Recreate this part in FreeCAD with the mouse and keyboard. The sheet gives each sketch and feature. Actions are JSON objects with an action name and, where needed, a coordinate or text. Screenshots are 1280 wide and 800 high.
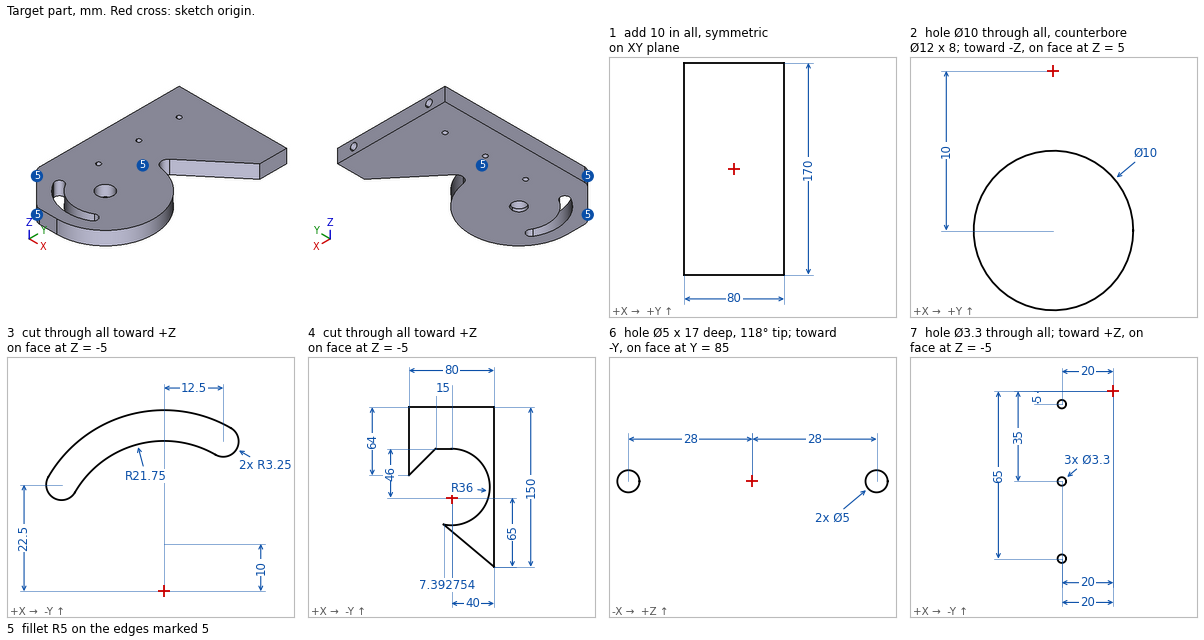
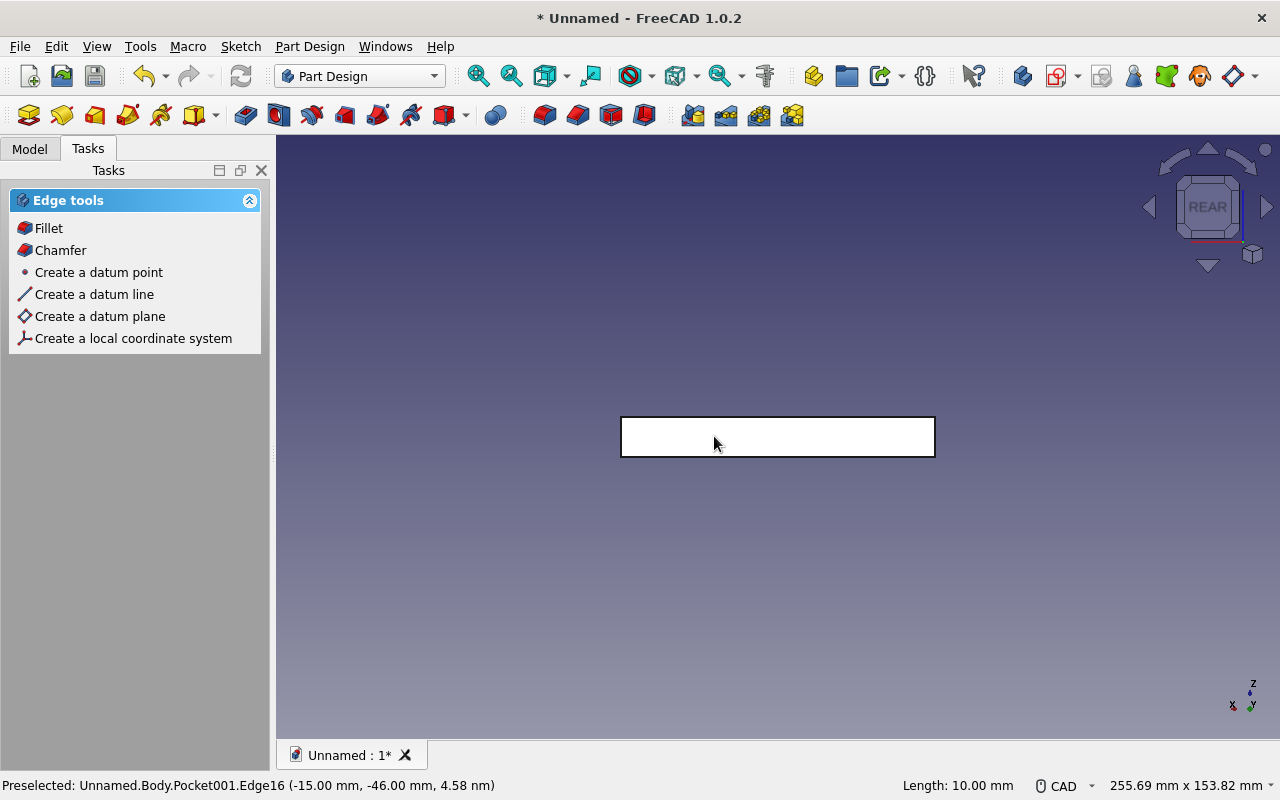
{"action": "key", "text": "6"}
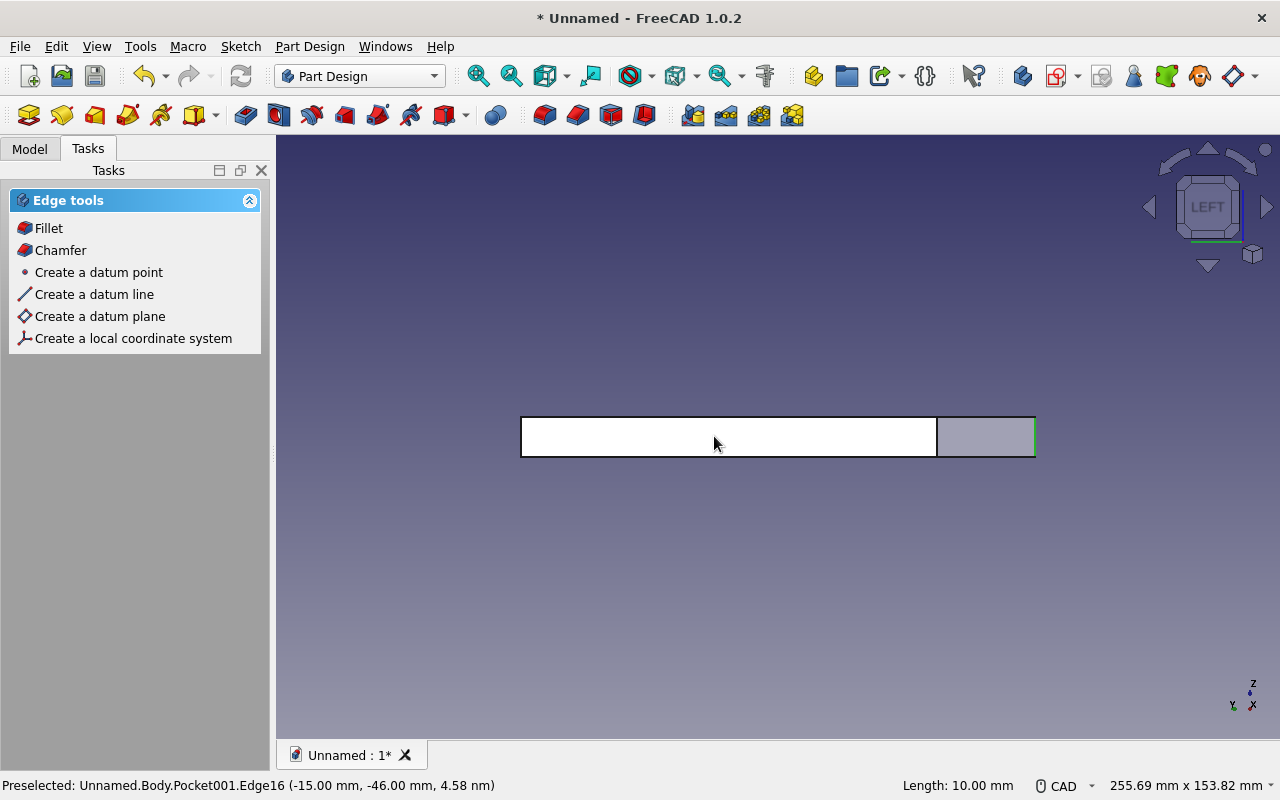
{"action": "left_click", "coordinate": [937, 436], "text": "ctrl"}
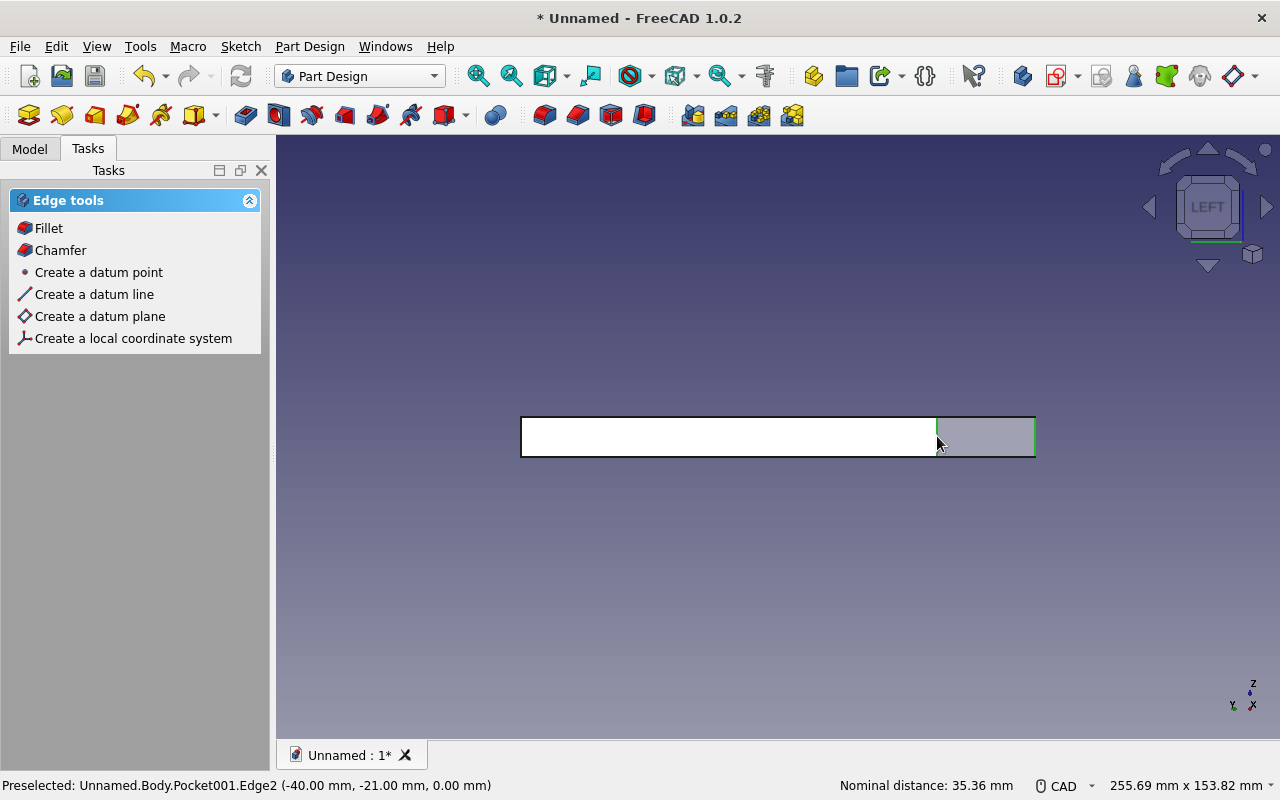
{"action": "key", "text": "v 3"}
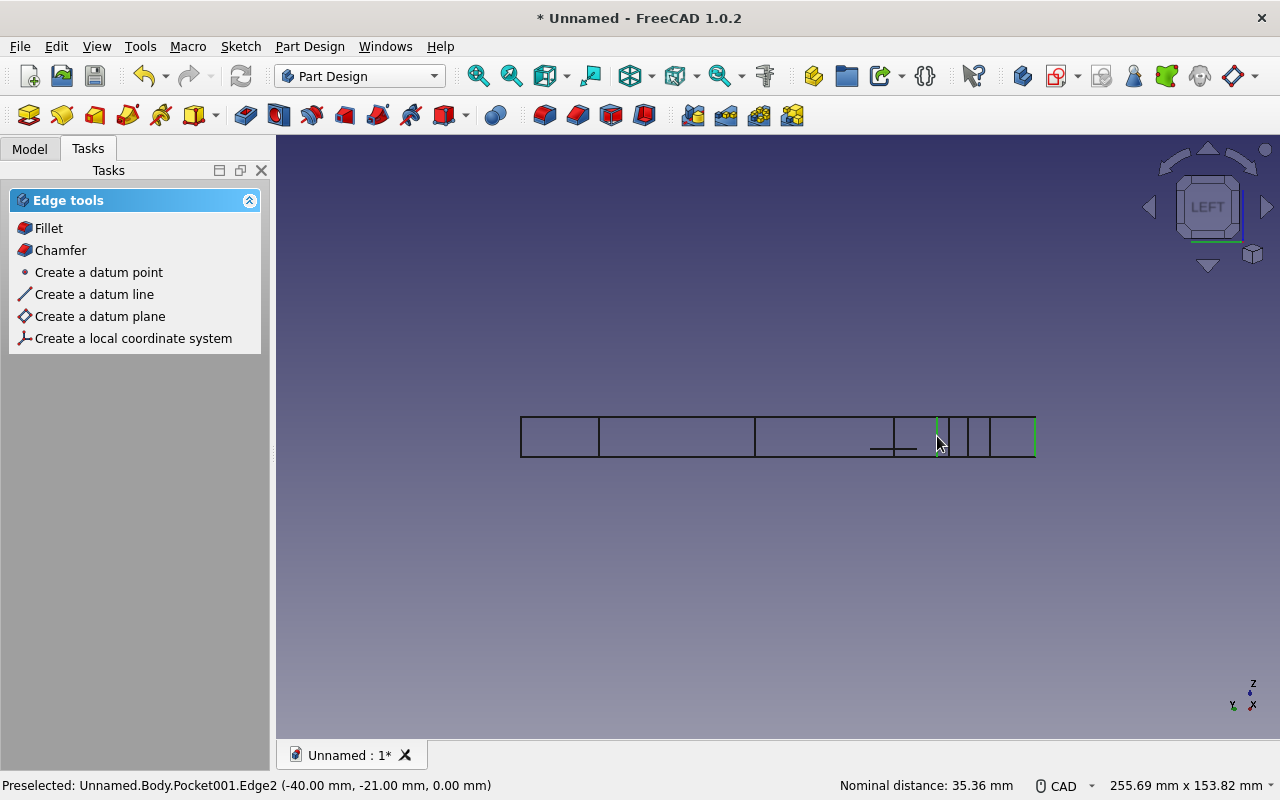
{"action": "key", "text": "0"}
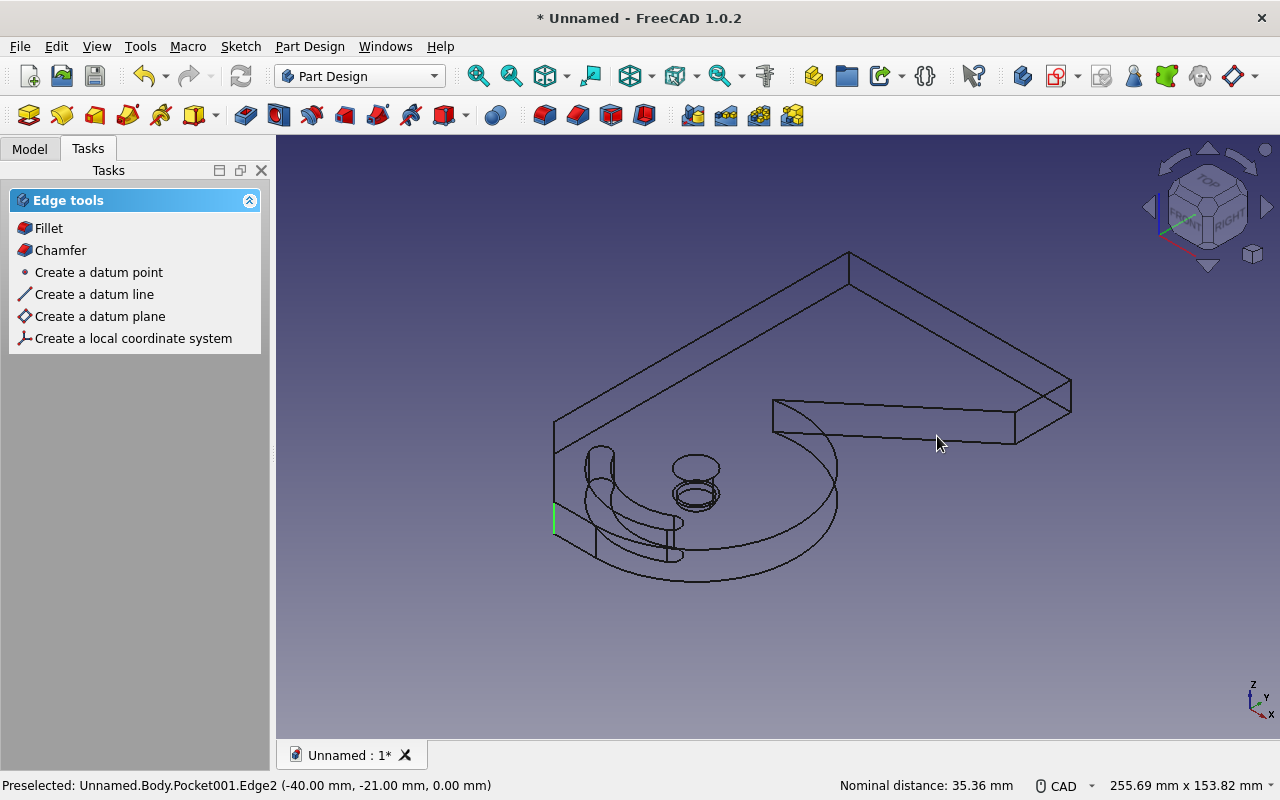
{"action": "left_click", "coordinate": [773, 415], "text": "ctrl"}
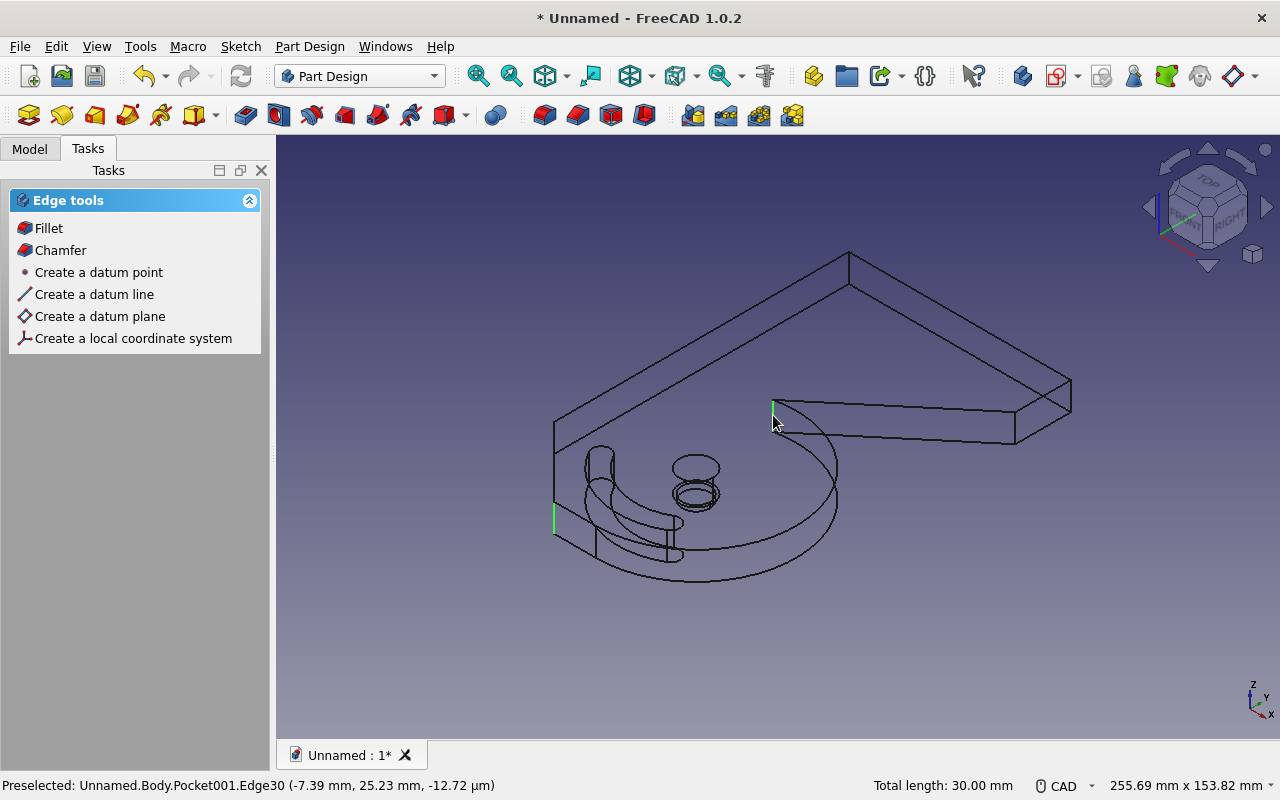
{"action": "key", "text": "v 1"}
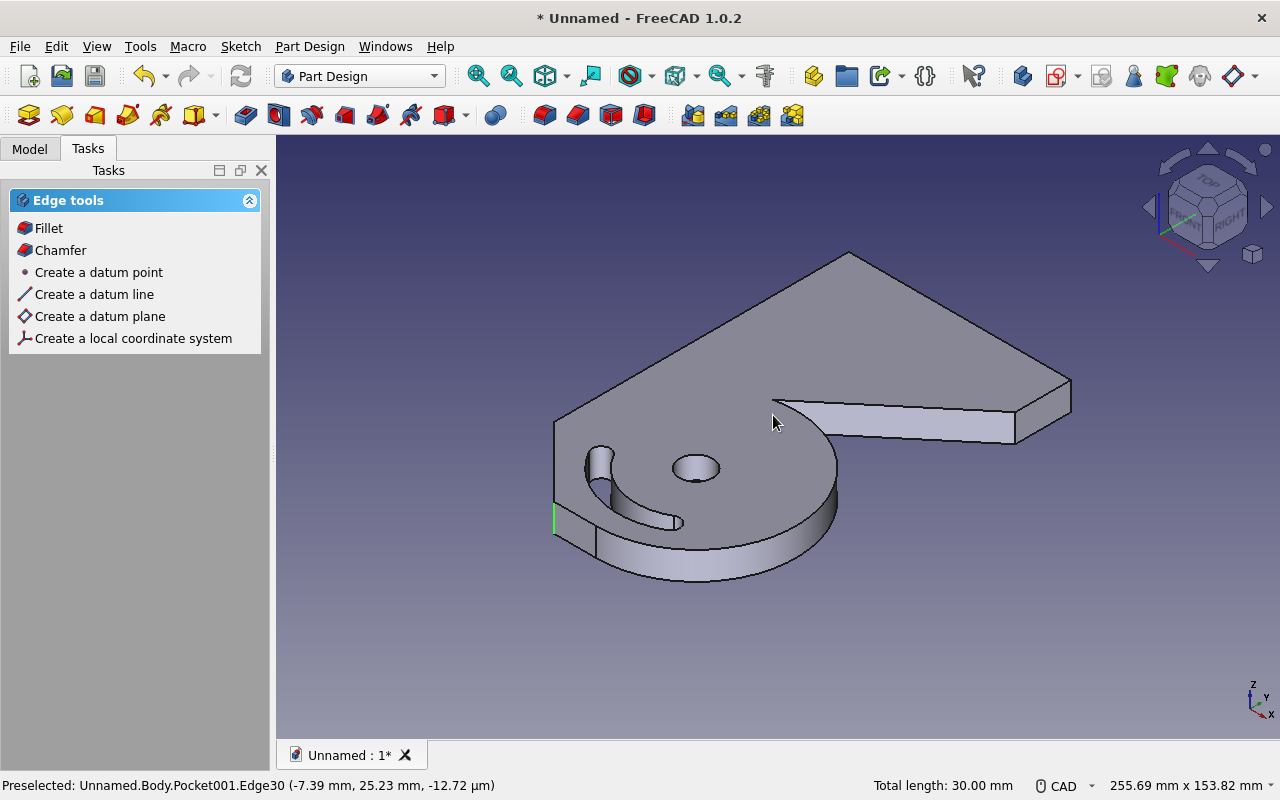
{"action": "left_click", "coordinate": [545, 116]}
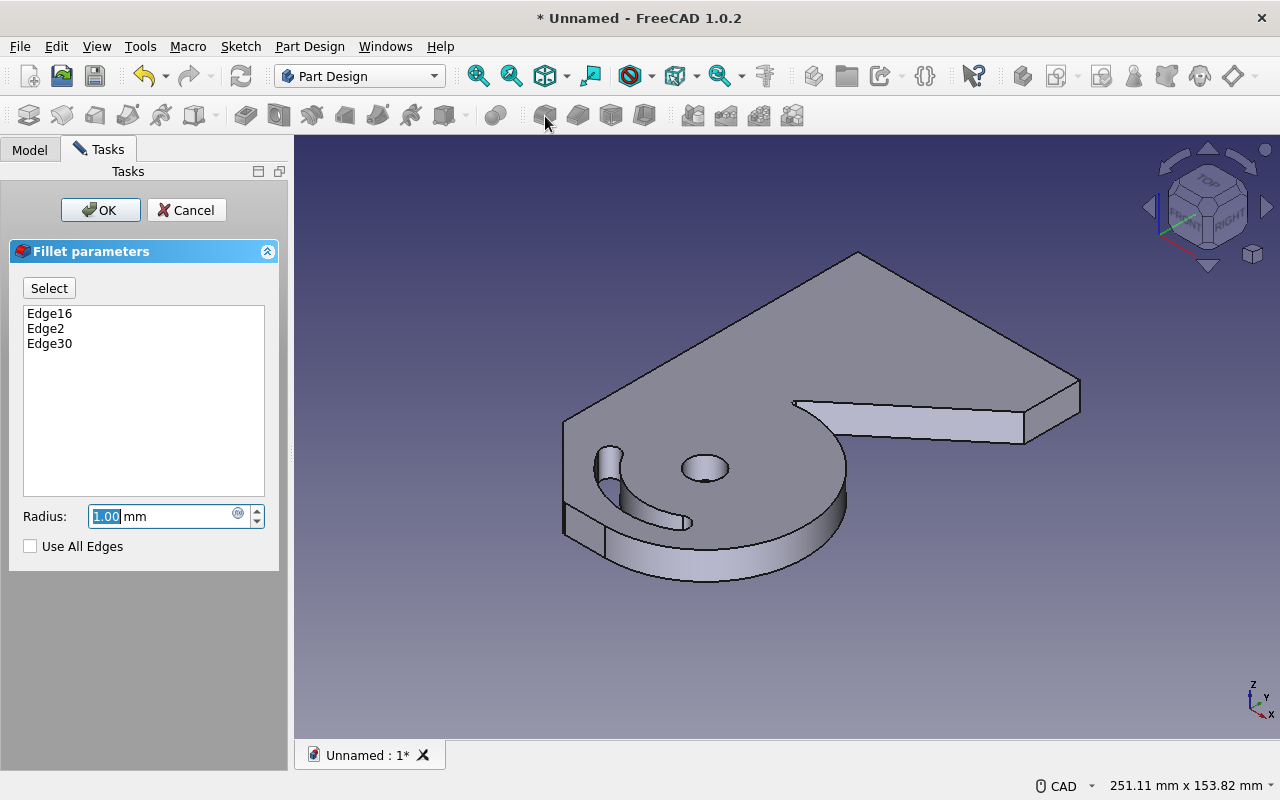
{"action": "type", "text": "5"}
{"action": "key", "text": "Tab"}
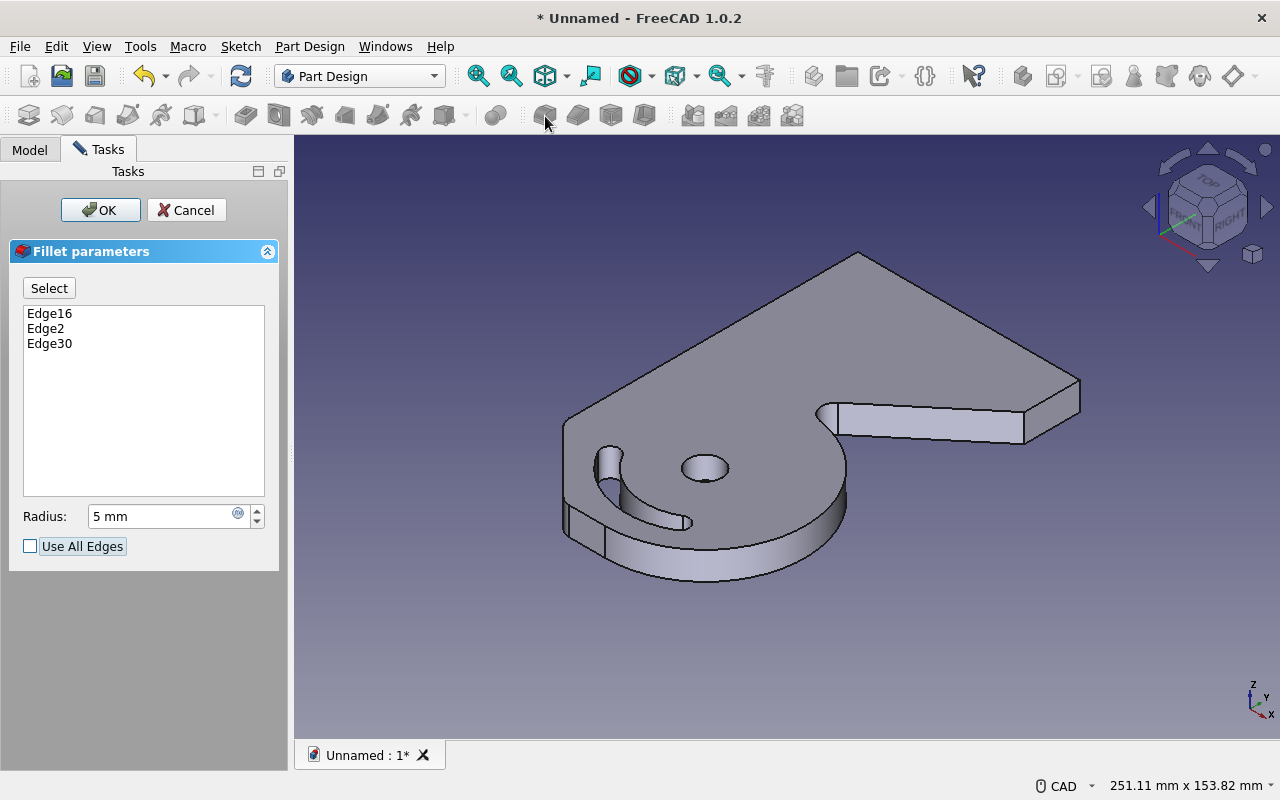
{"action": "left_click", "coordinate": [101, 210]}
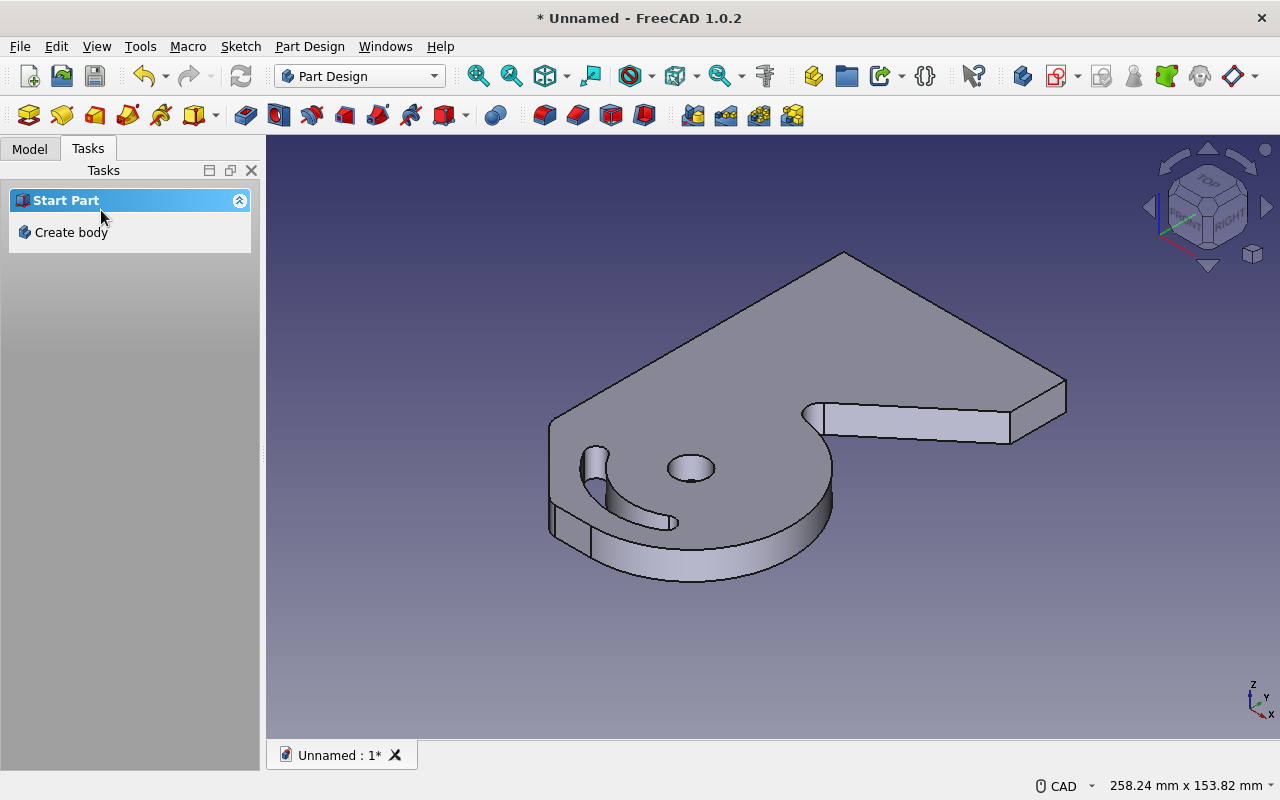
{"action": "key", "text": "4"}